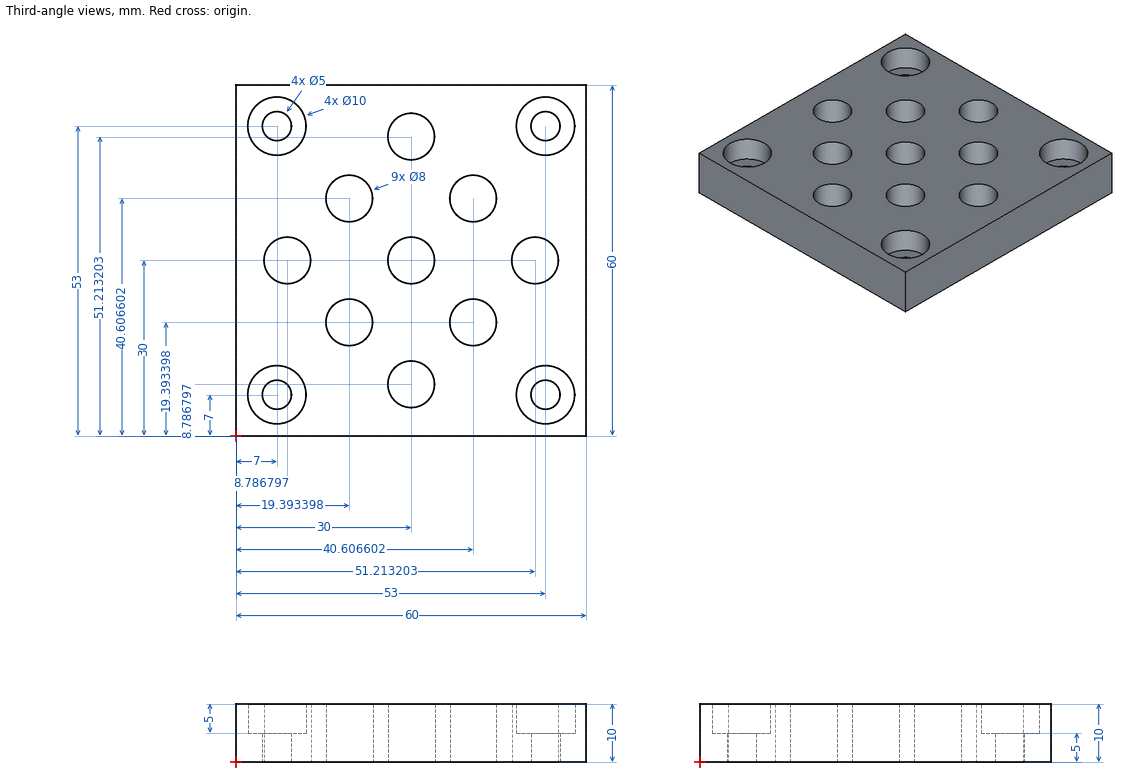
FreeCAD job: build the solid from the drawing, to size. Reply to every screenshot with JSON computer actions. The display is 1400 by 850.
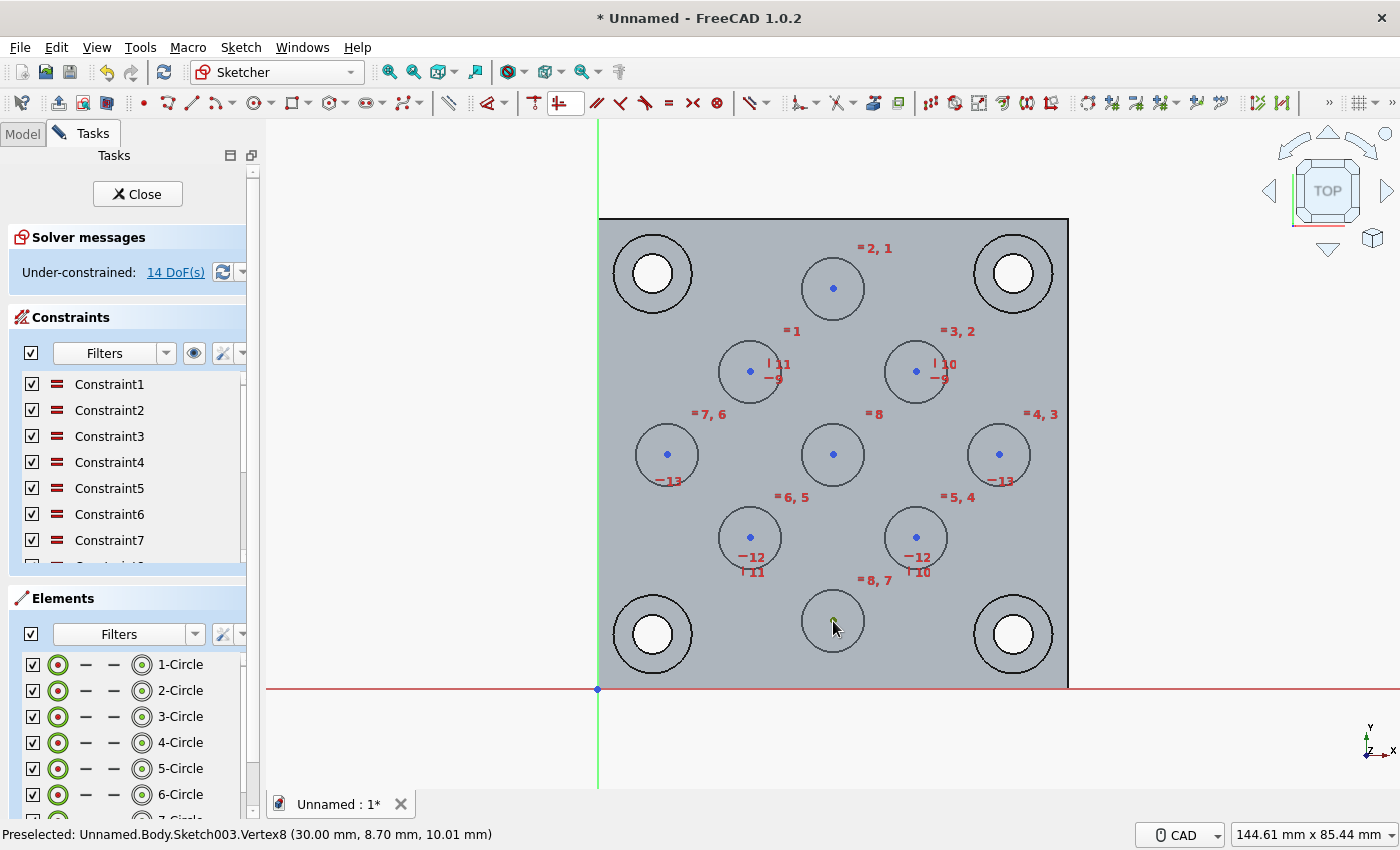
{"action": "left_click", "coordinate": [833, 455]}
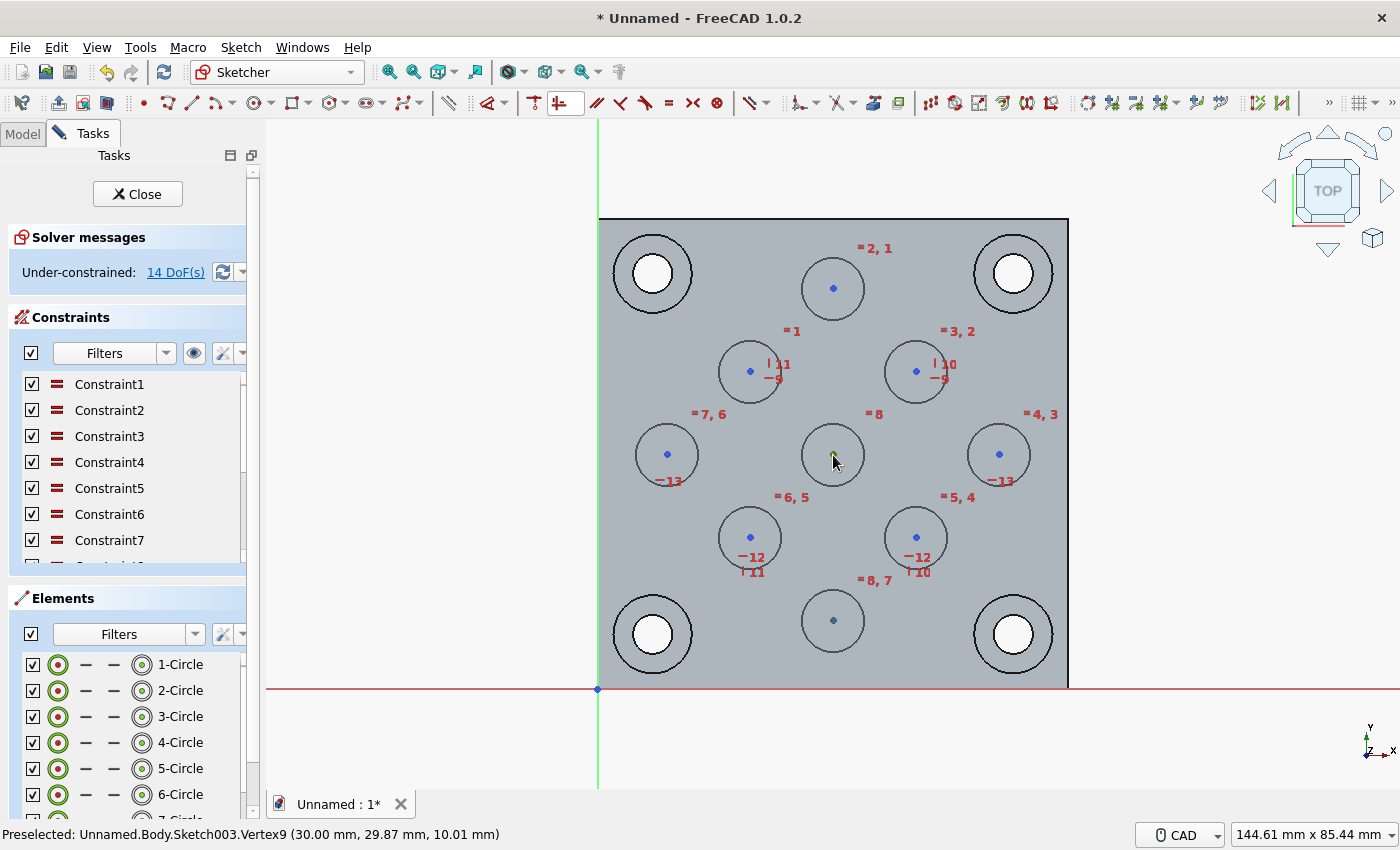
{"action": "left_click", "coordinate": [578, 104]}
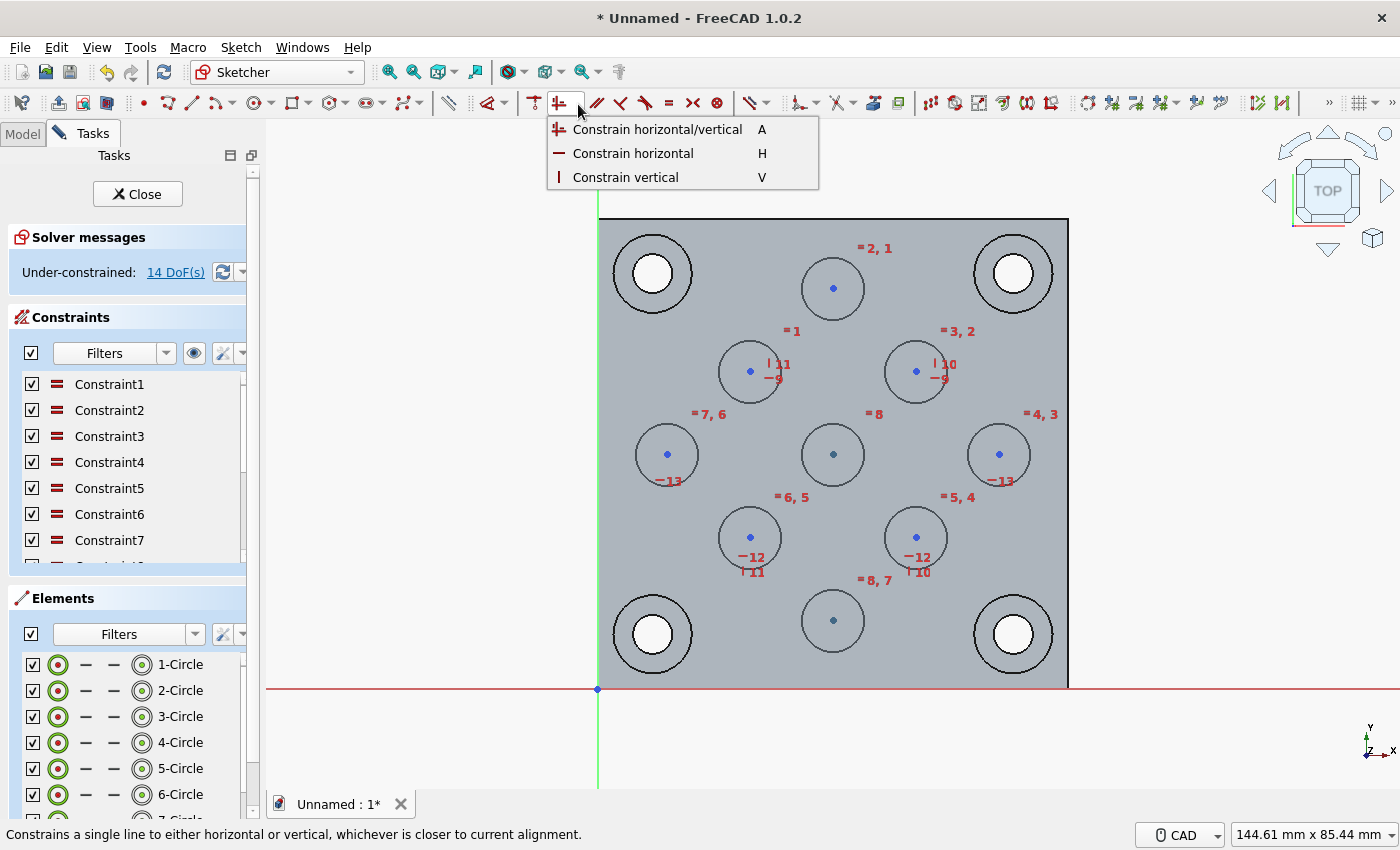
{"action": "left_click", "coordinate": [683, 177]}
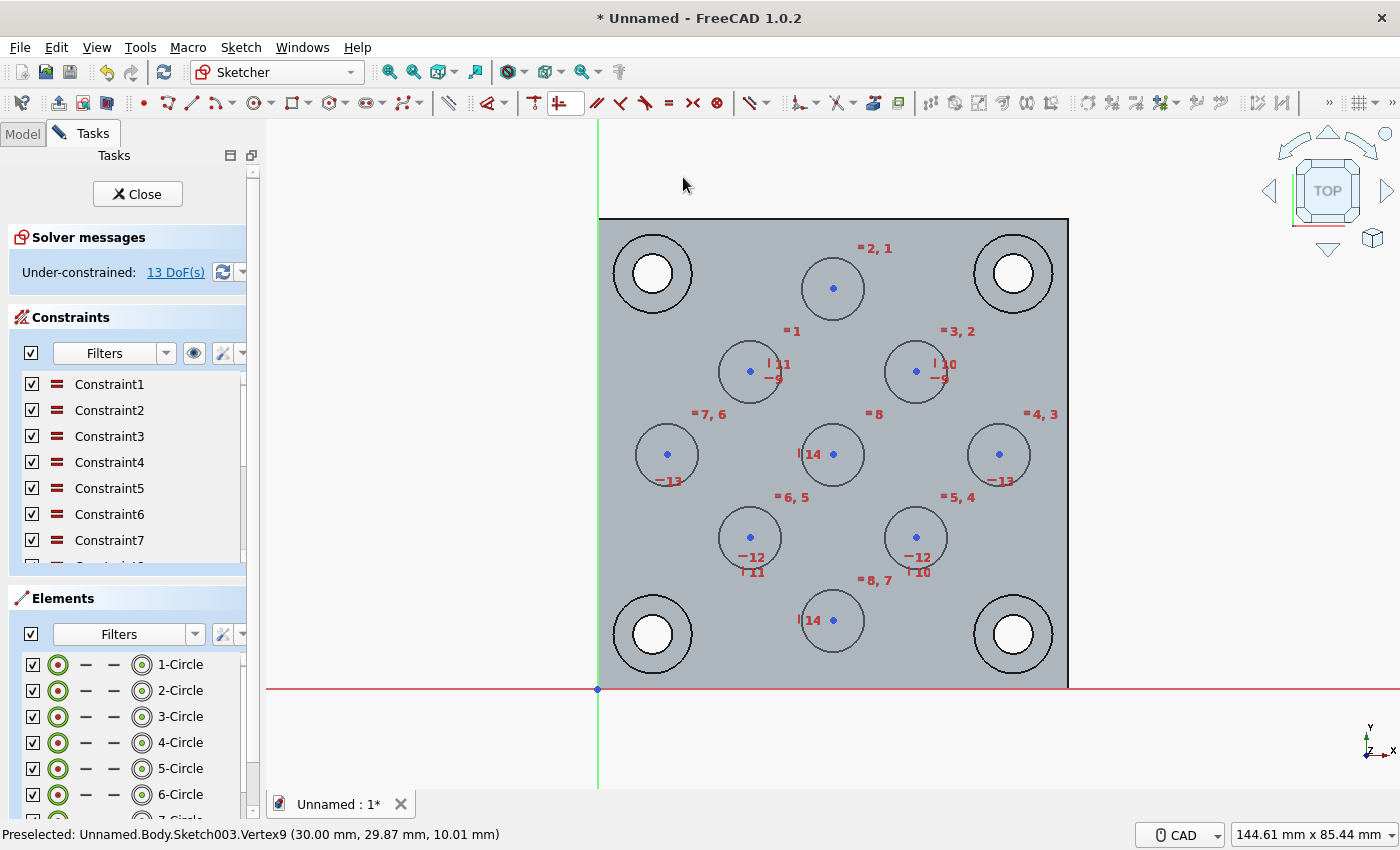
{"action": "left_click", "coordinate": [667, 455]}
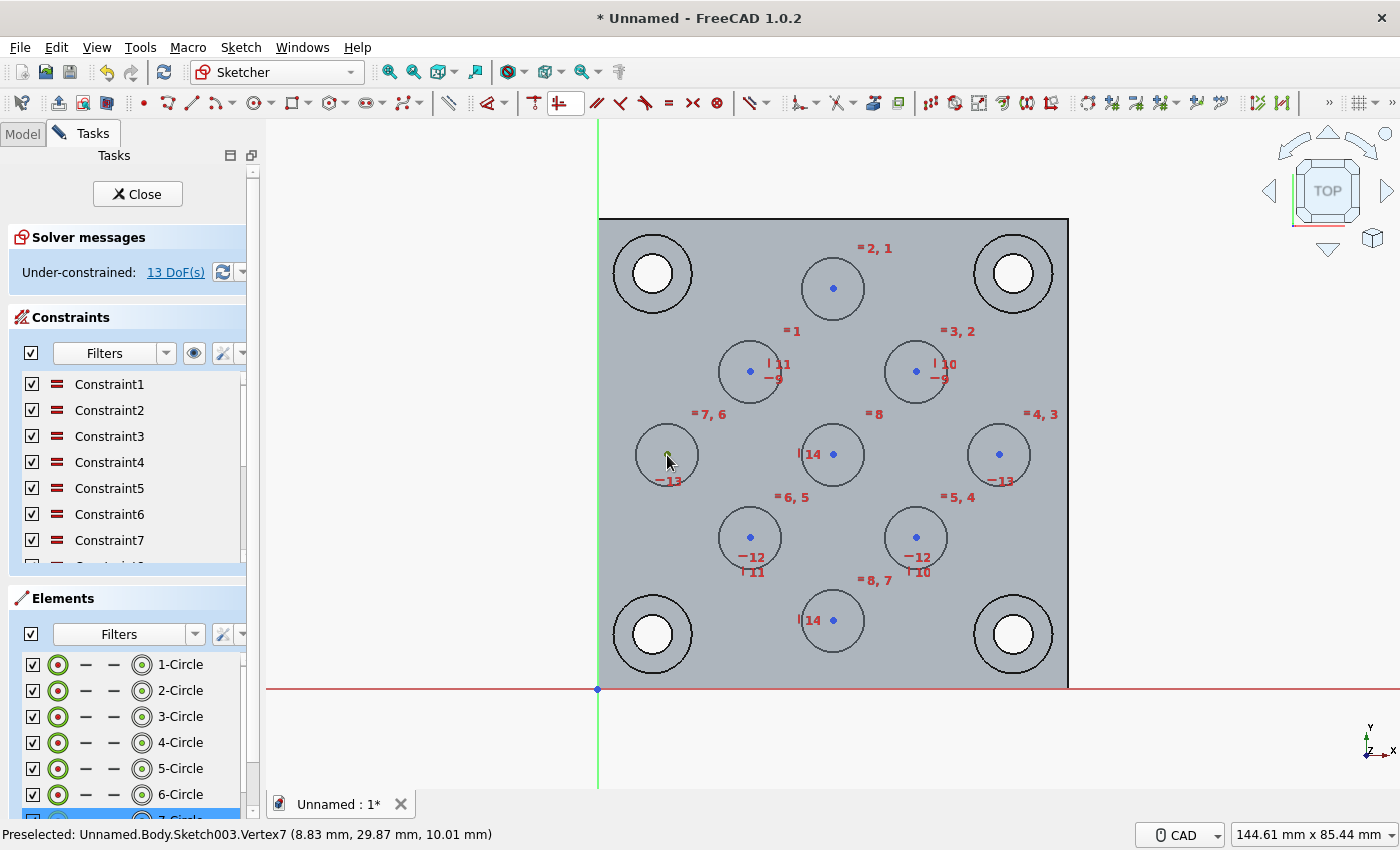
{"action": "left_click", "coordinate": [833, 455]}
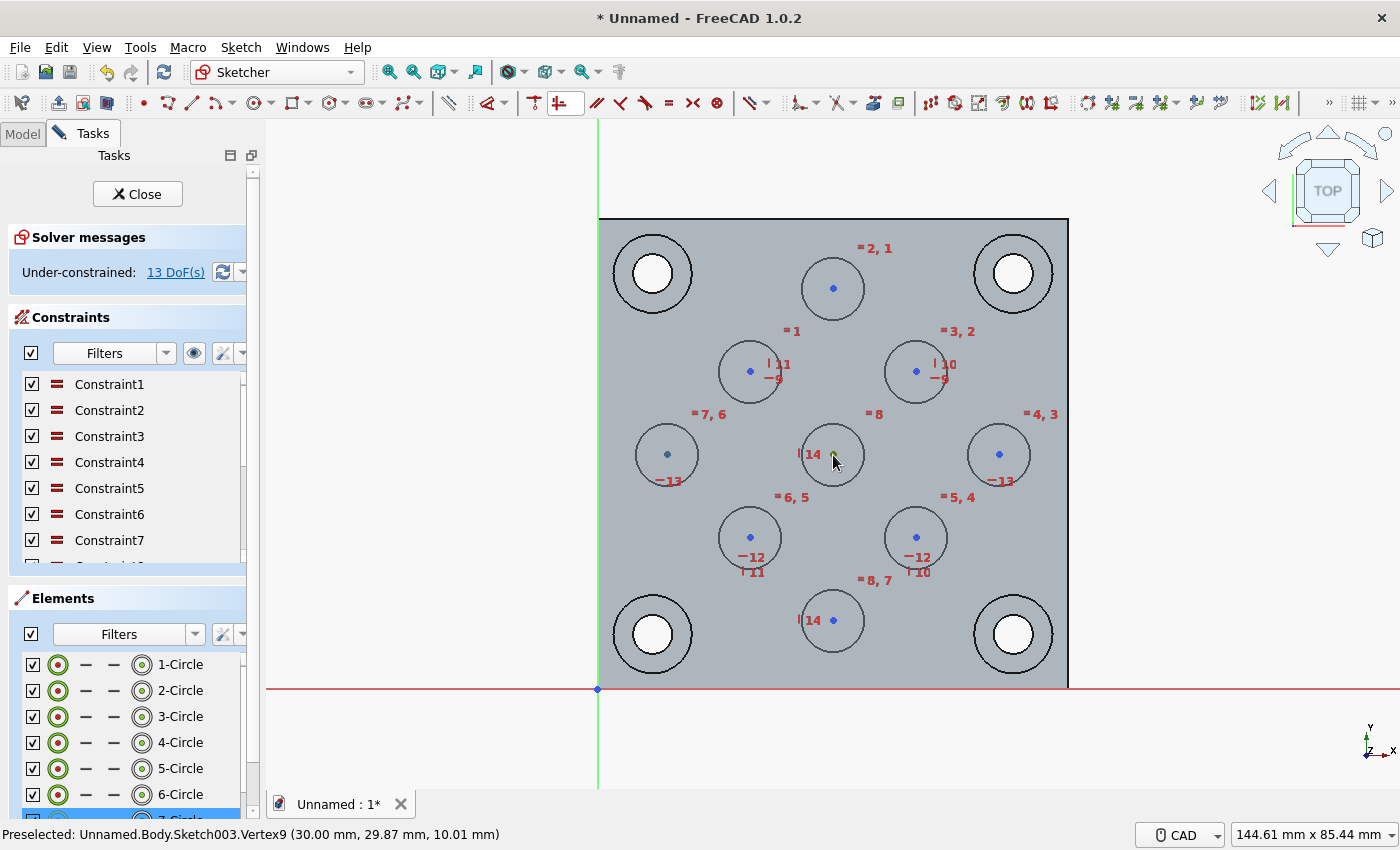
{"action": "key", "text": "h"}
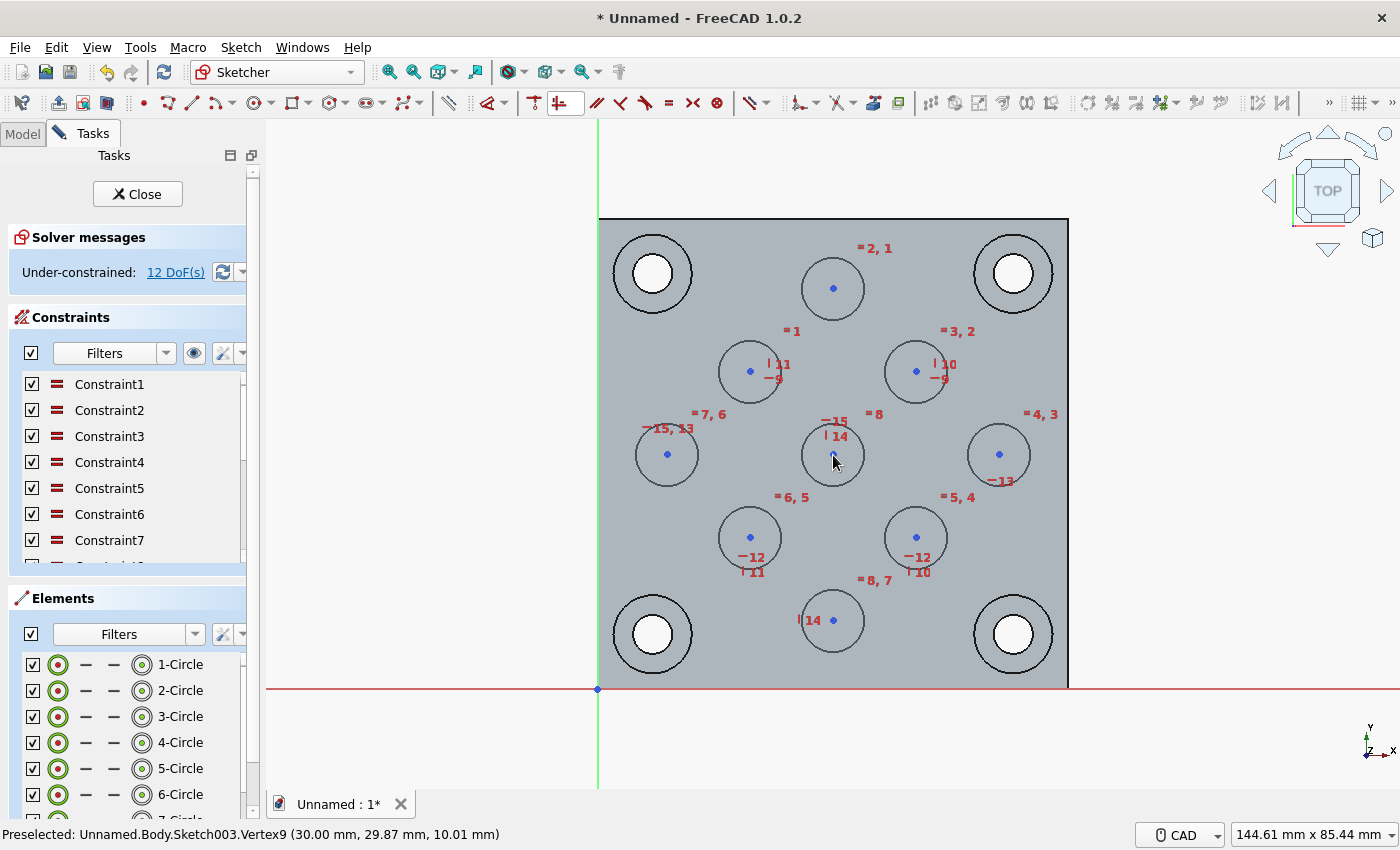
{"action": "key", "text": "d"}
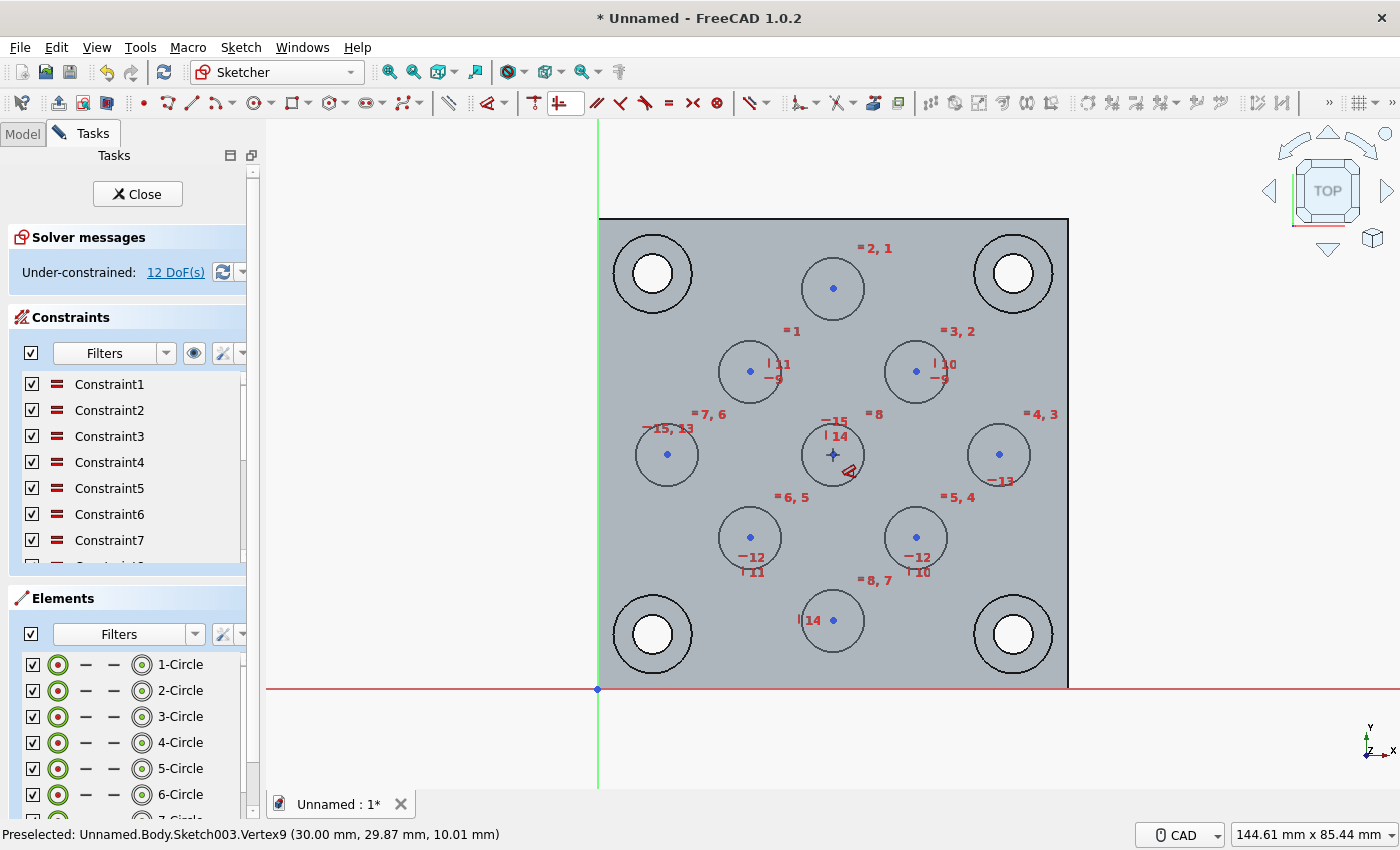
{"action": "left_click", "coordinate": [772, 350]}
{"action": "left_click", "coordinate": [795, 327]}